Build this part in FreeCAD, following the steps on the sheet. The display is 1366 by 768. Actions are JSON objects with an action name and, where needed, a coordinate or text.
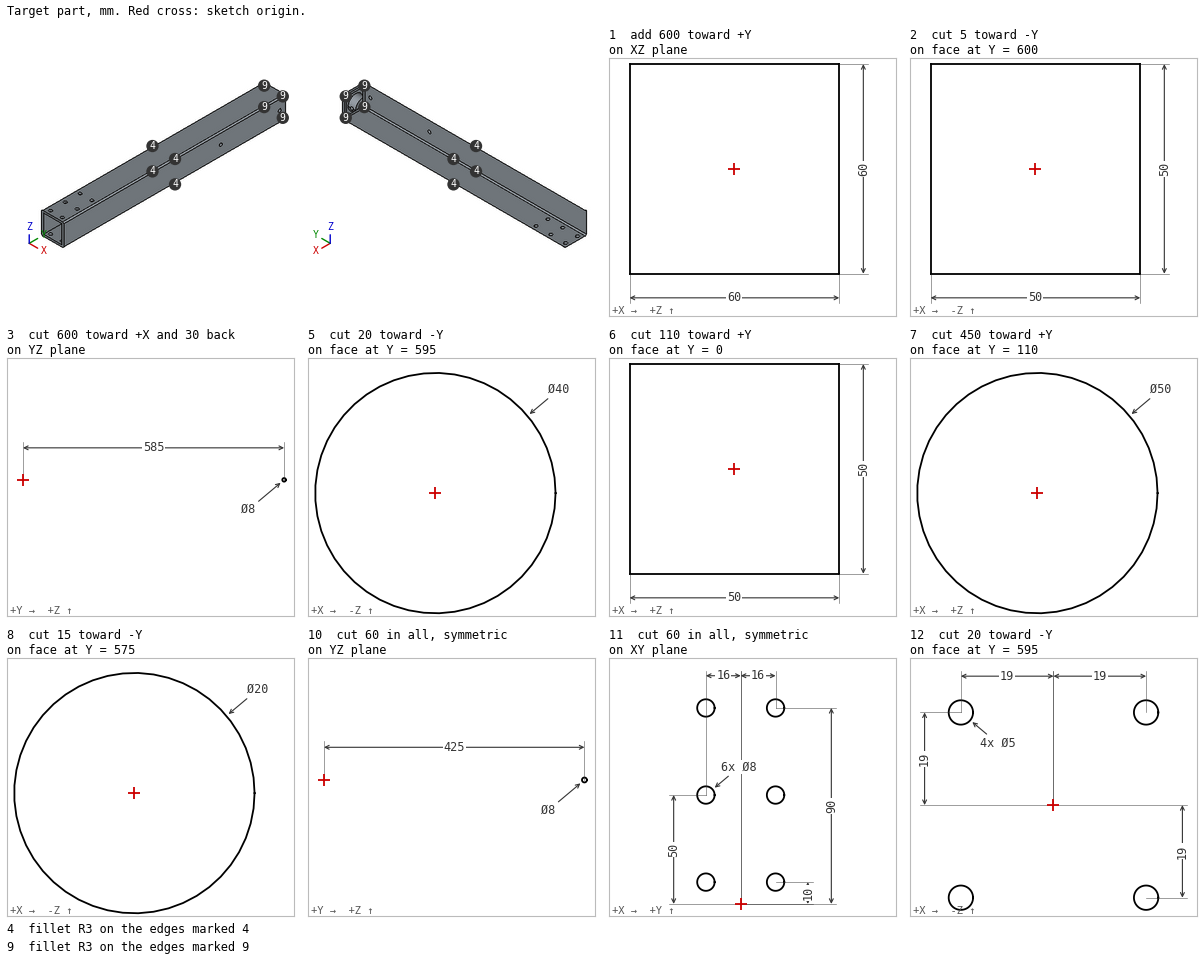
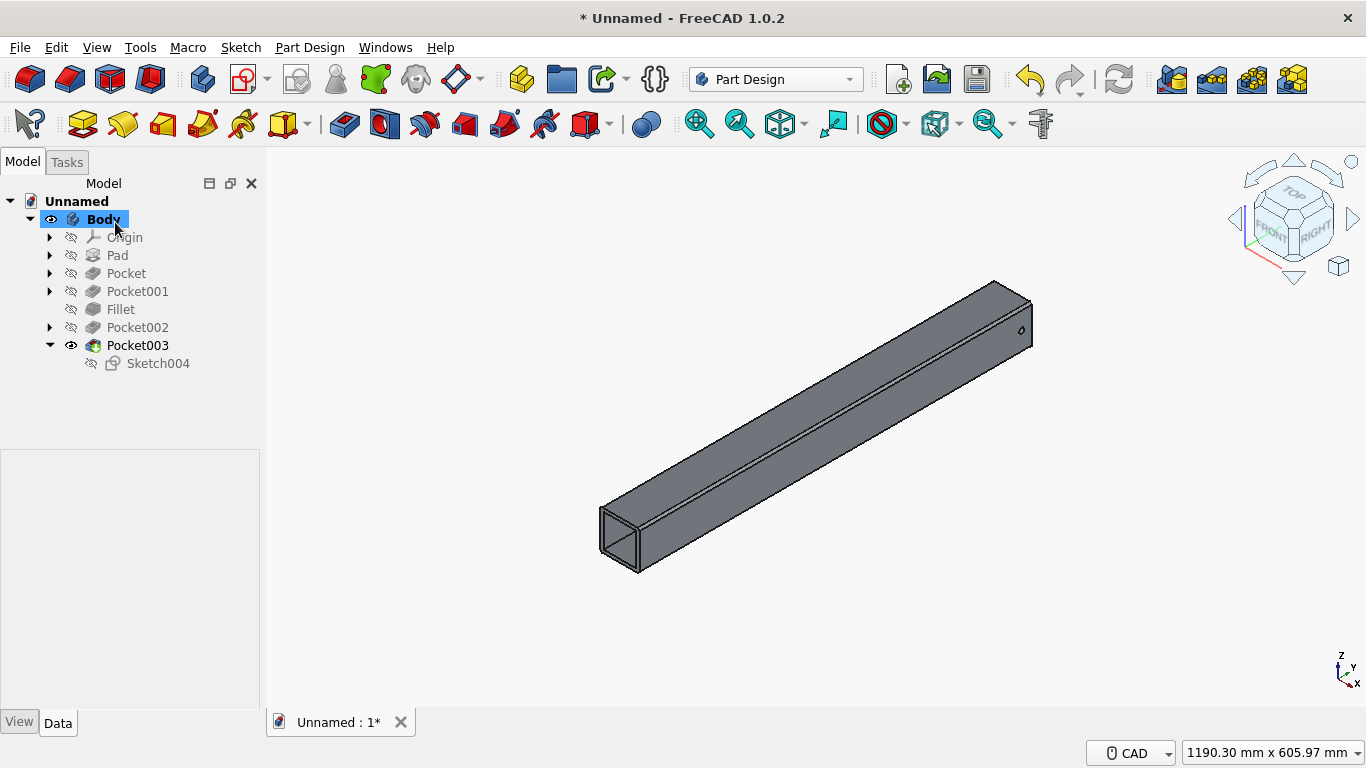
{"action": "key", "text": "1"}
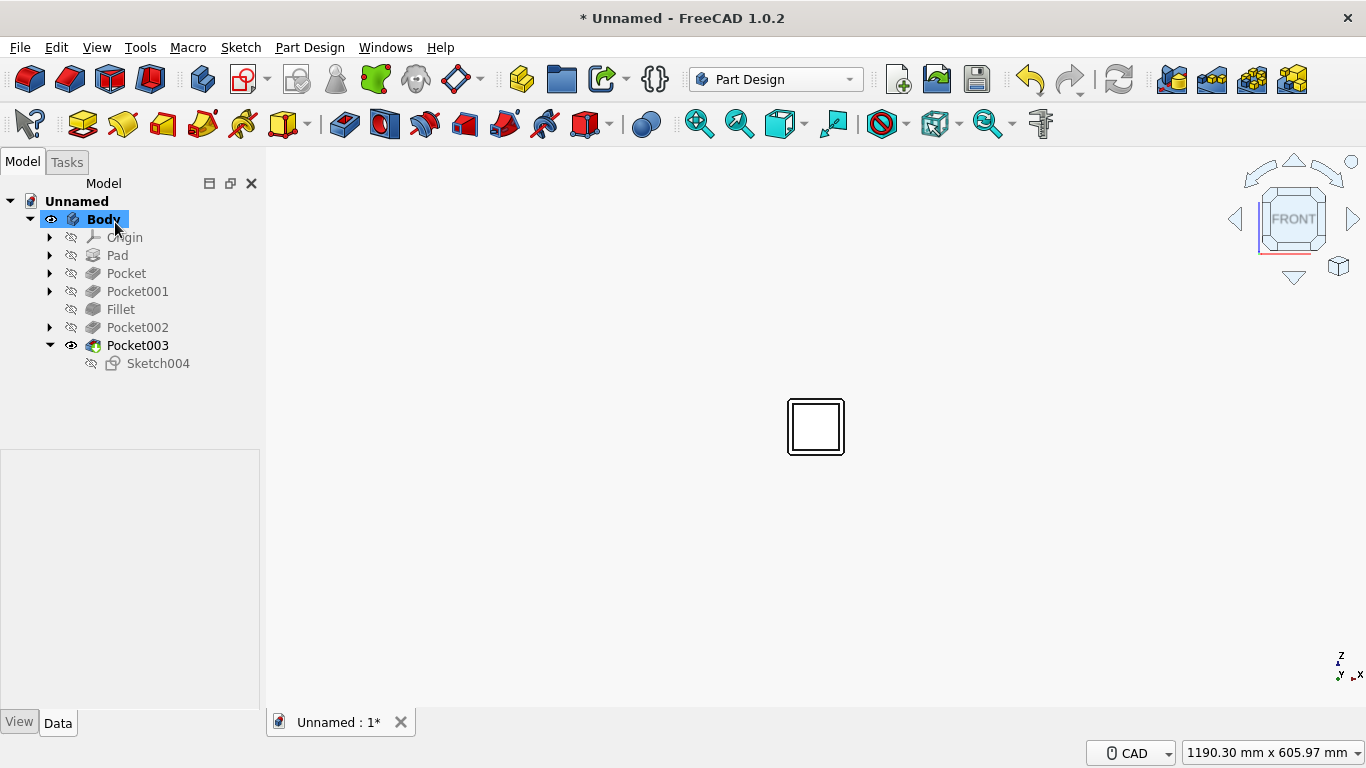
{"action": "left_click", "coordinate": [700, 124]}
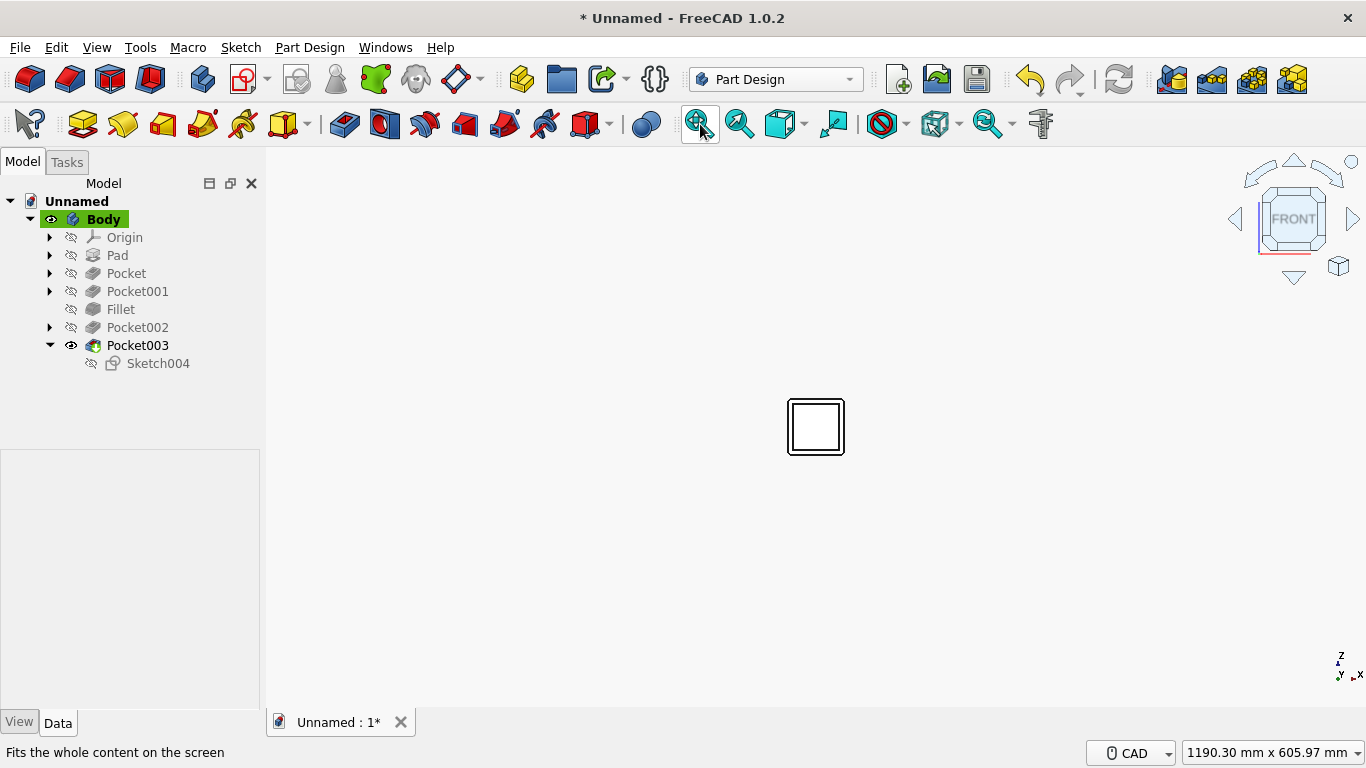
{"action": "left_click", "coordinate": [816, 426]}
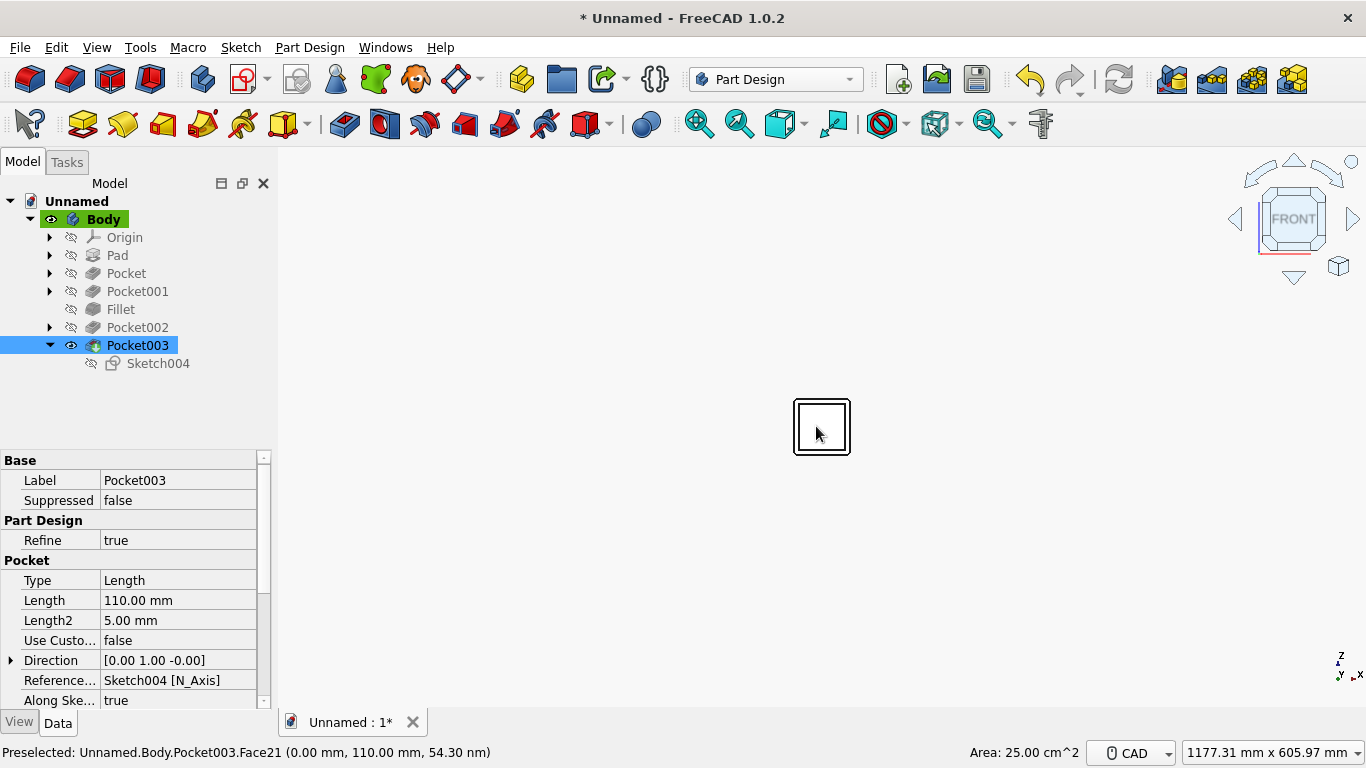
{"action": "left_click", "coordinate": [244, 80]}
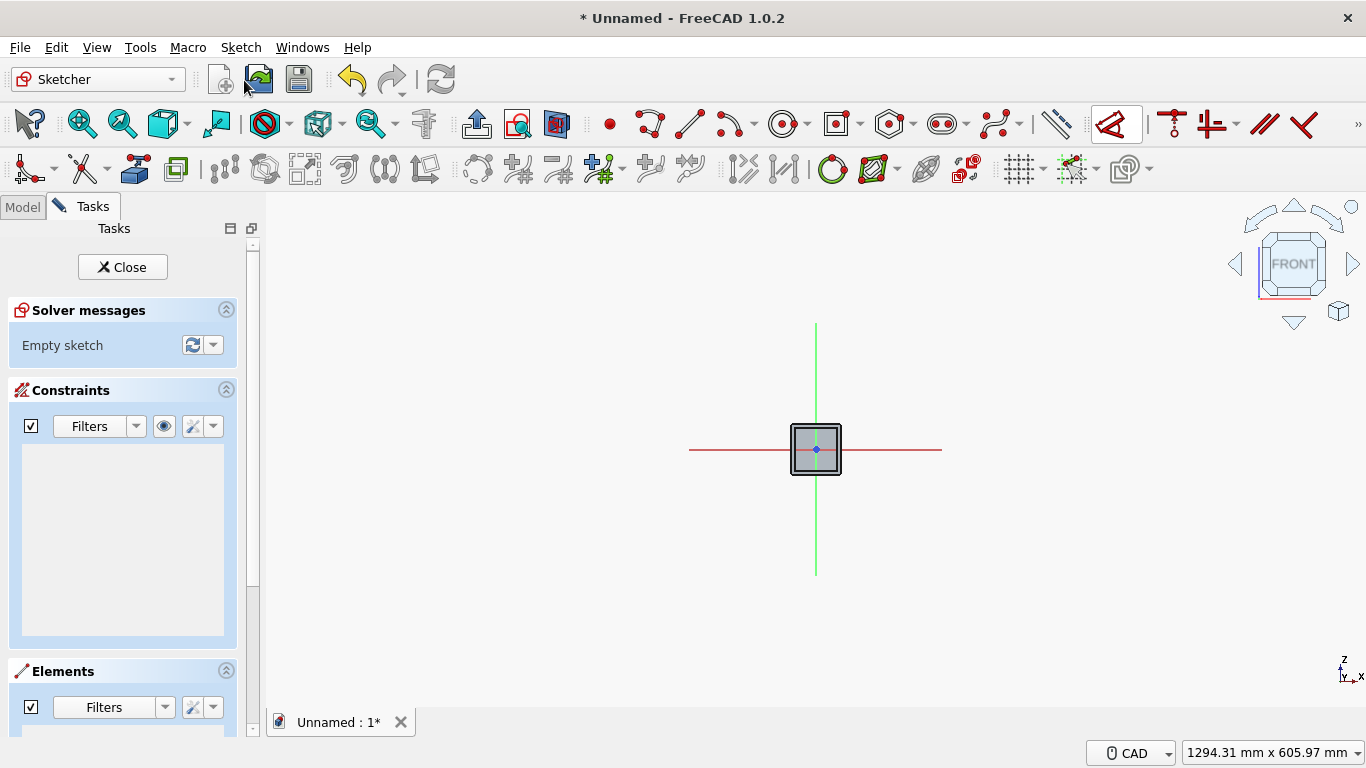
{"action": "key", "text": "q s"}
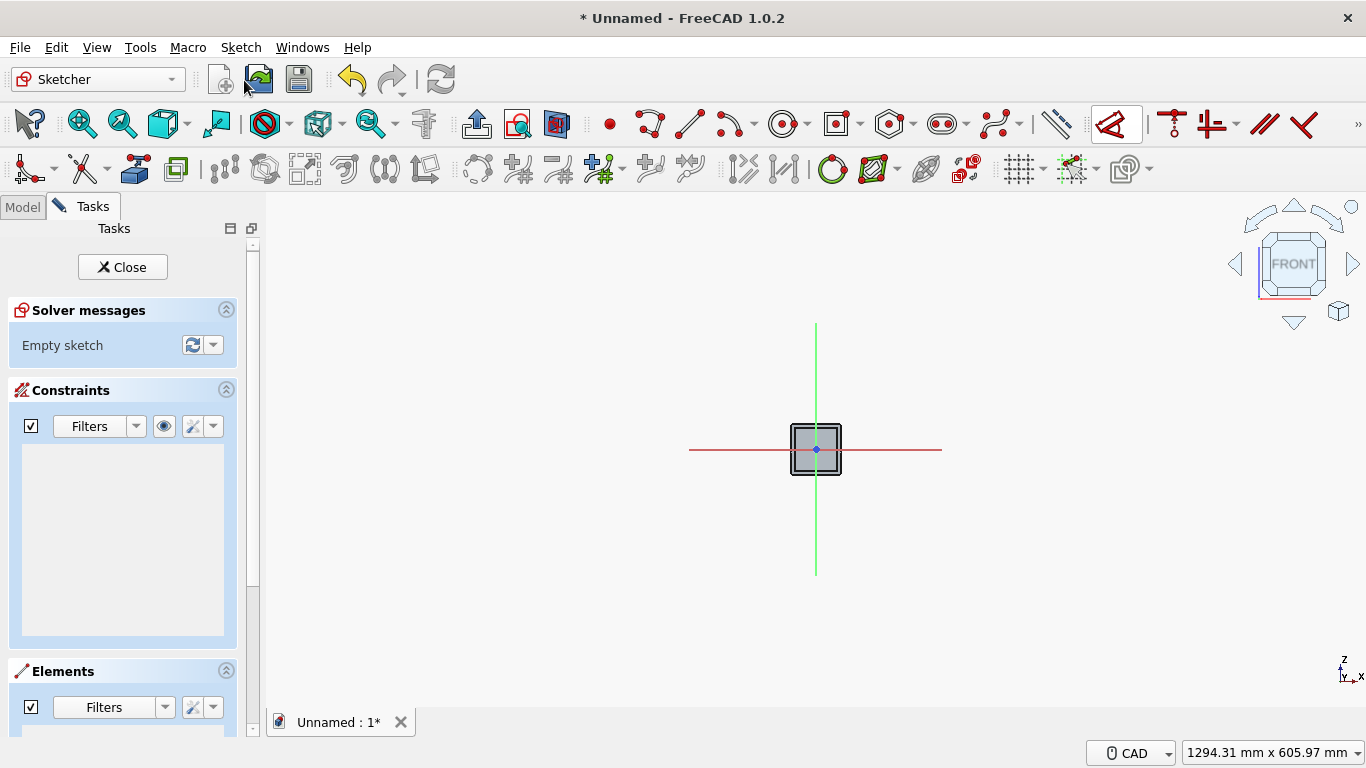
{"action": "scroll", "coordinate": [827, 450], "scroll_direction": "up", "scroll_amount": 10}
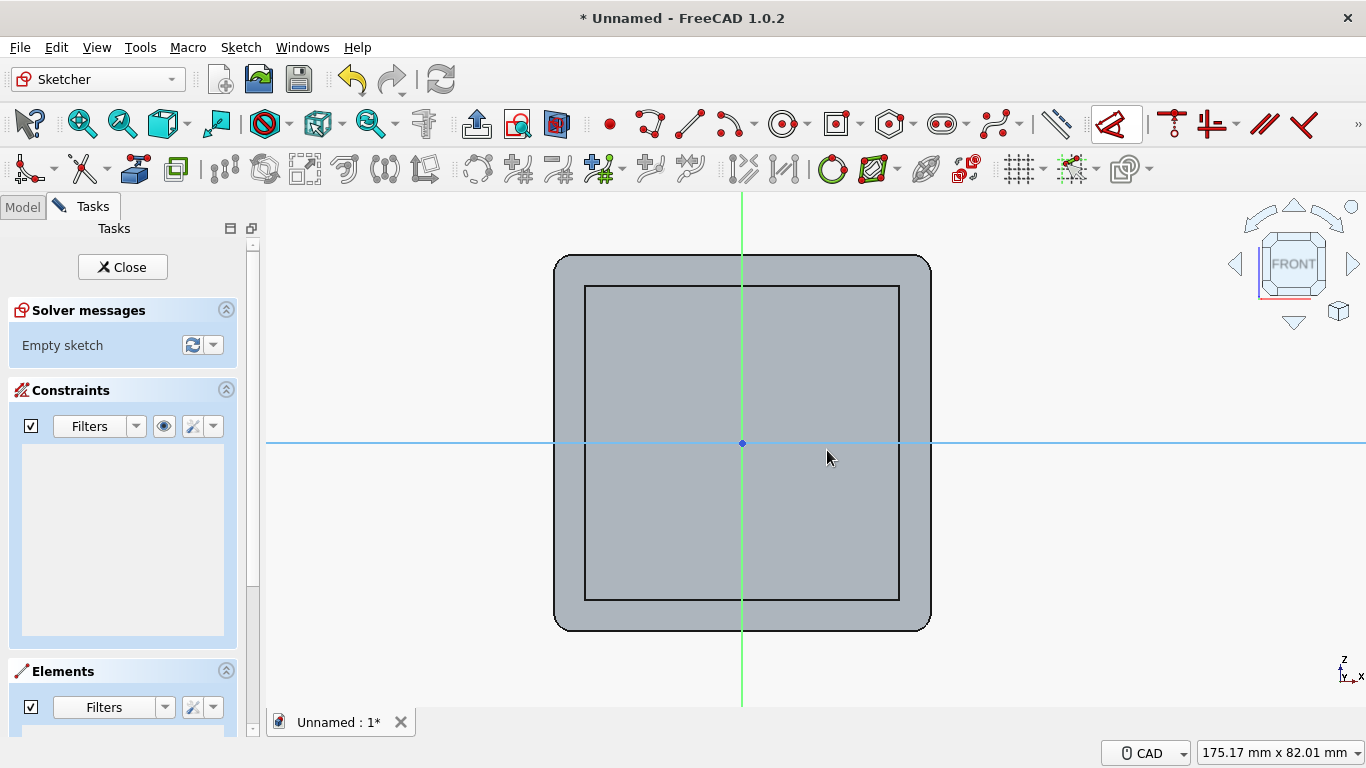
{"action": "left_click", "coordinate": [784, 124]}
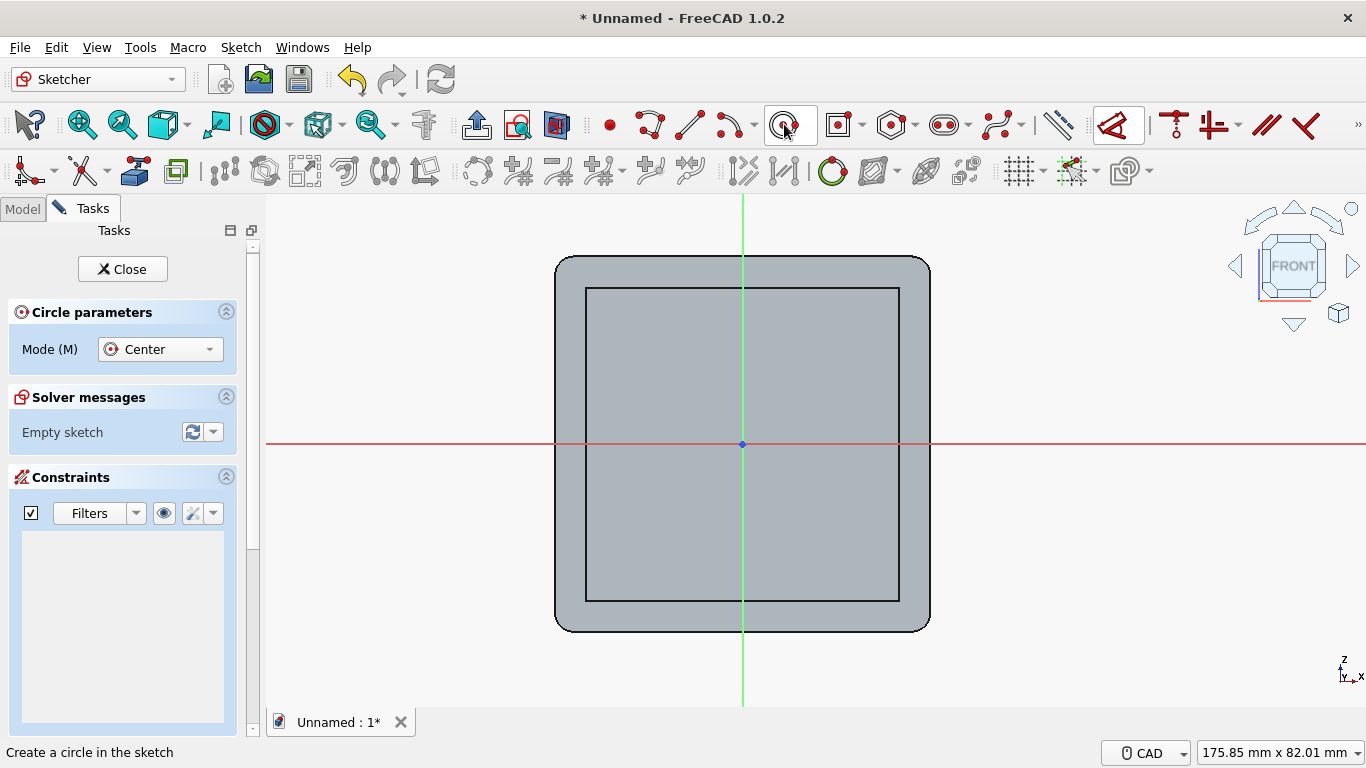
{"action": "left_click", "coordinate": [743, 444]}
{"action": "mouse_move", "coordinate": [853, 334]}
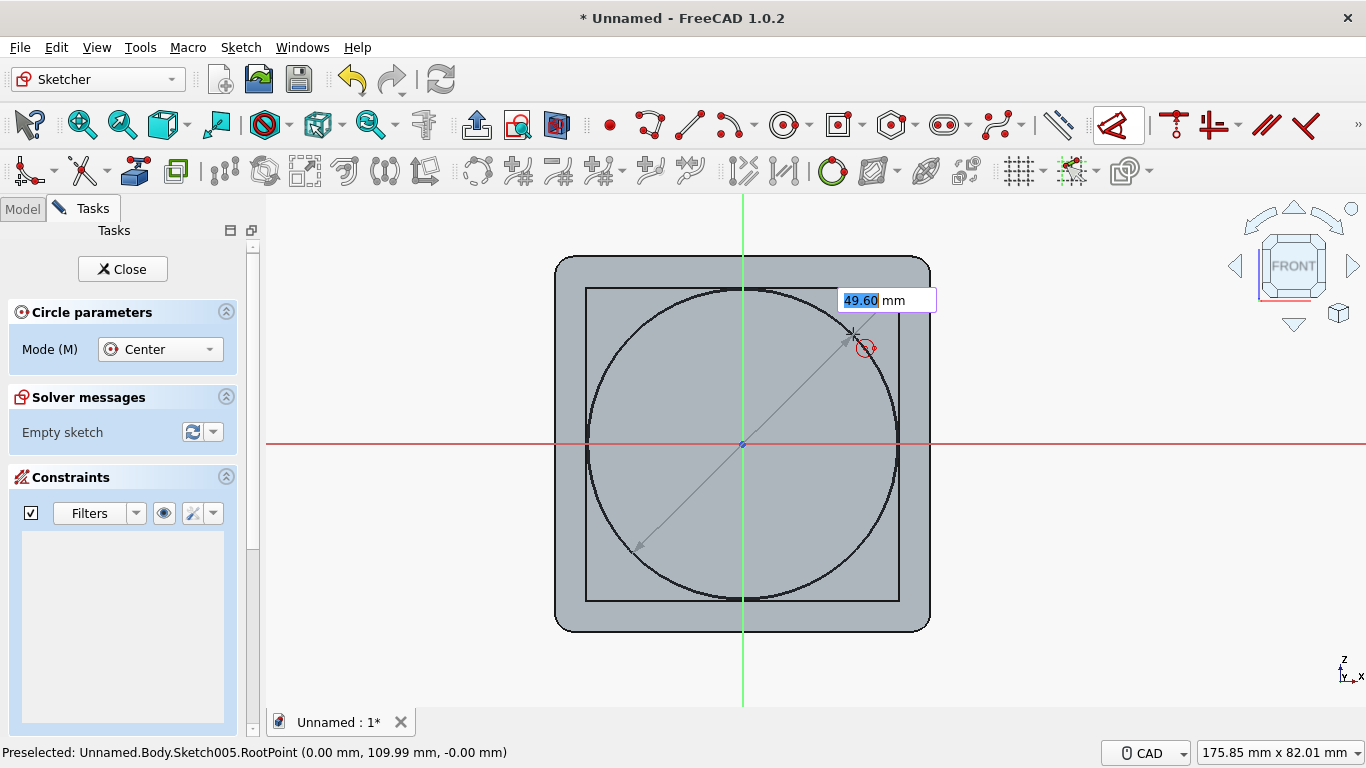
{"action": "type", "text": "50"}
{"action": "key", "text": "Return"}
{"action": "key", "text": "Escape"}